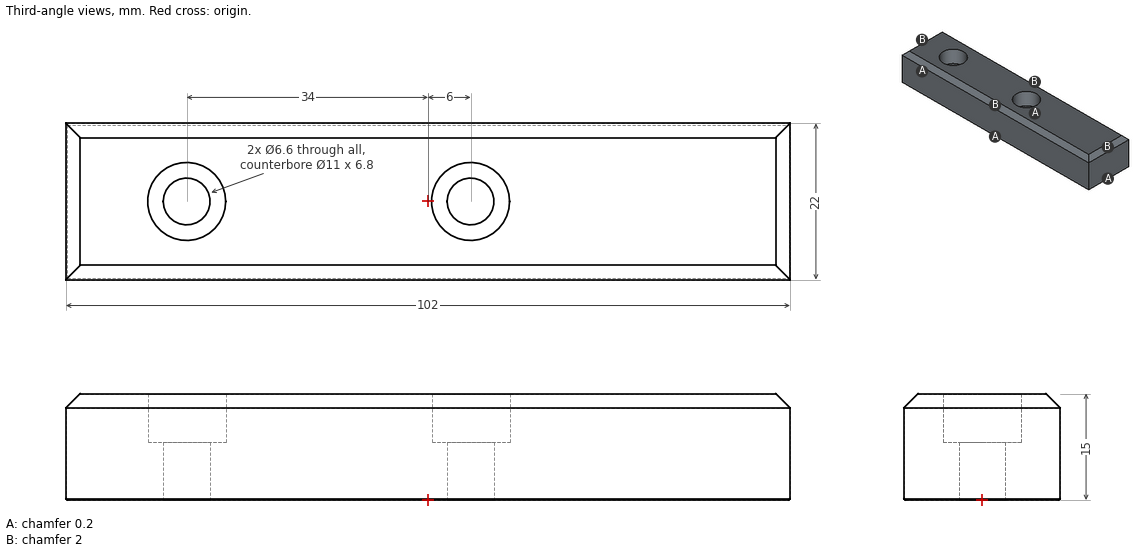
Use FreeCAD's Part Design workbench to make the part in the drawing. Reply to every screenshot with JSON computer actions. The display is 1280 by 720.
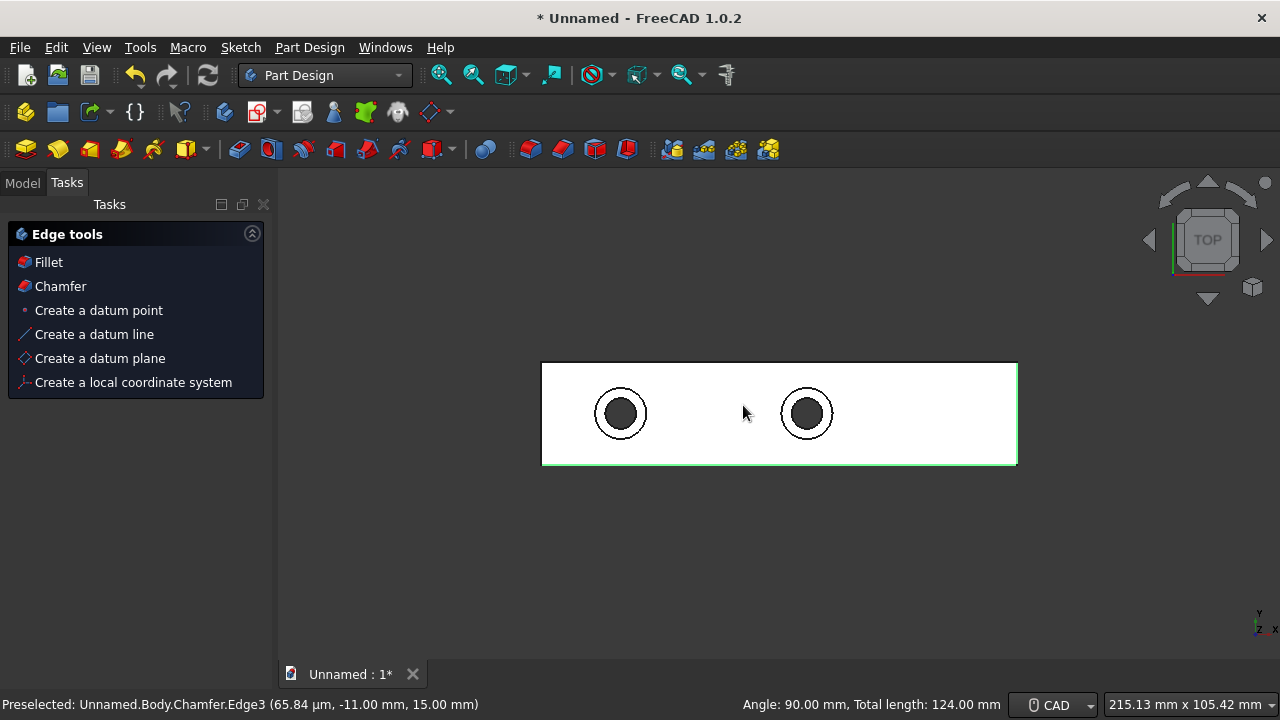
{"action": "left_click", "coordinate": [779, 361], "text": "ctrl"}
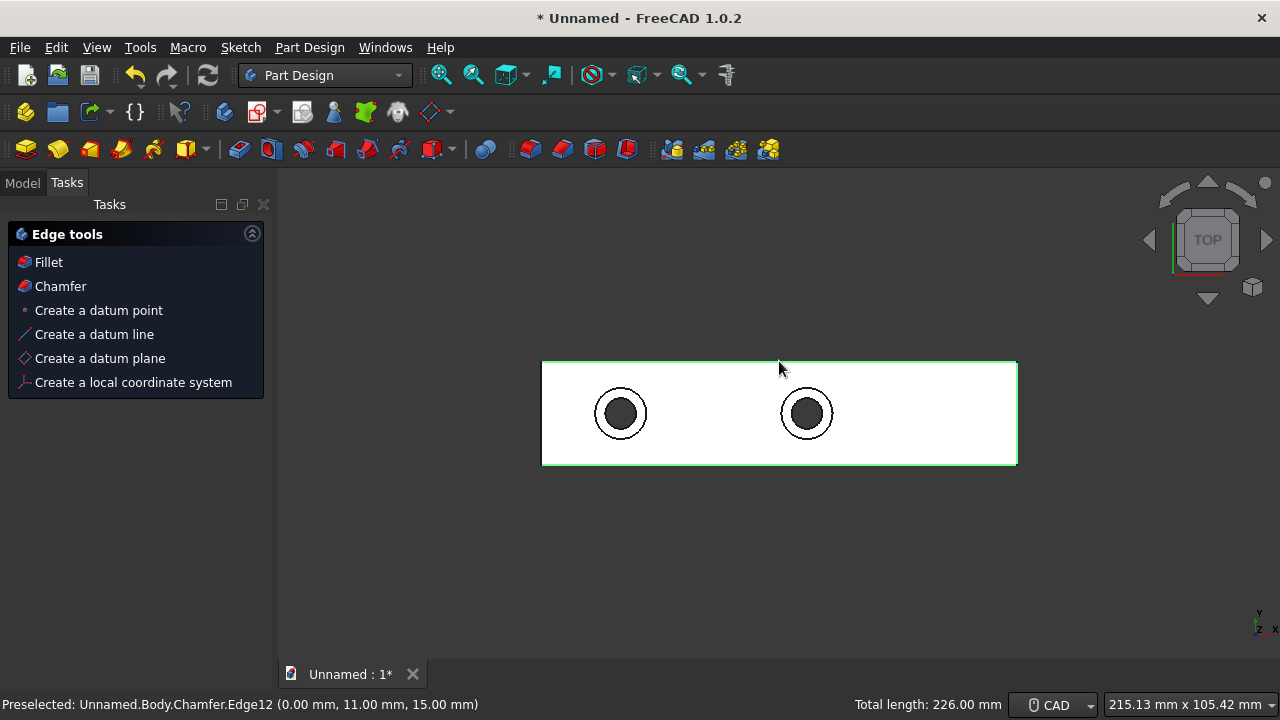
{"action": "left_click", "coordinate": [541, 413], "text": "ctrl"}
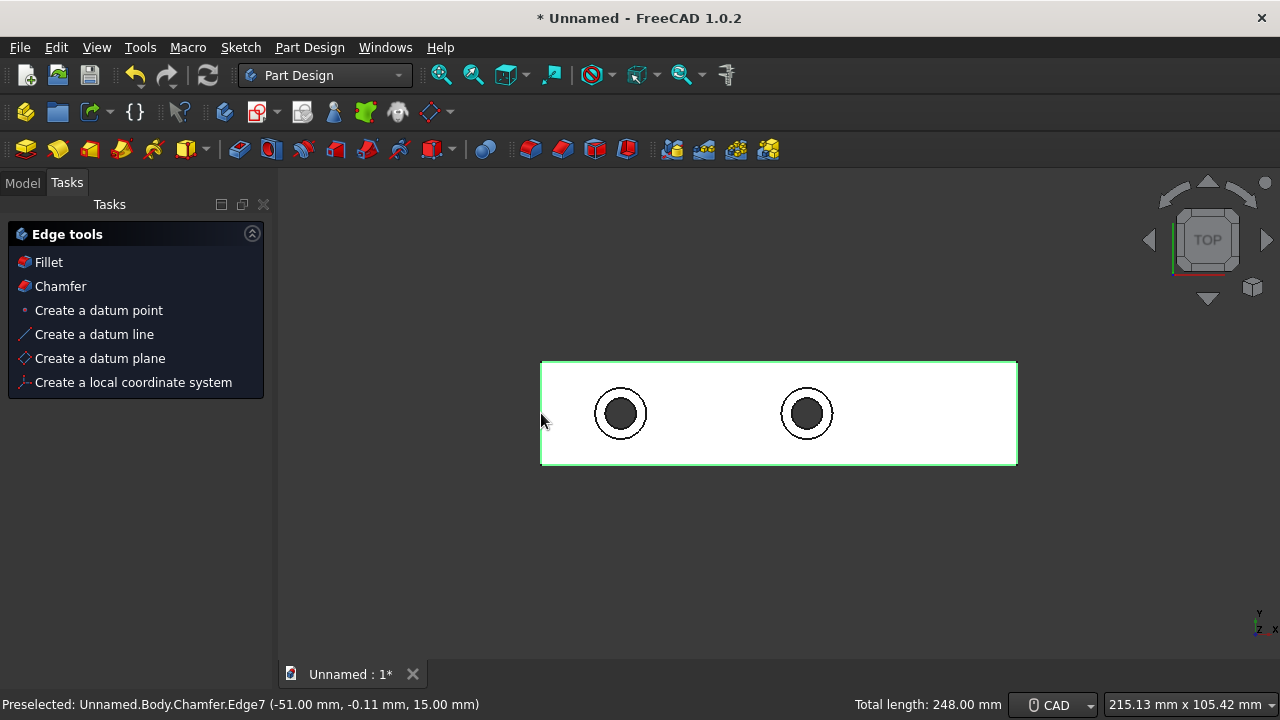
{"action": "left_click", "coordinate": [564, 150]}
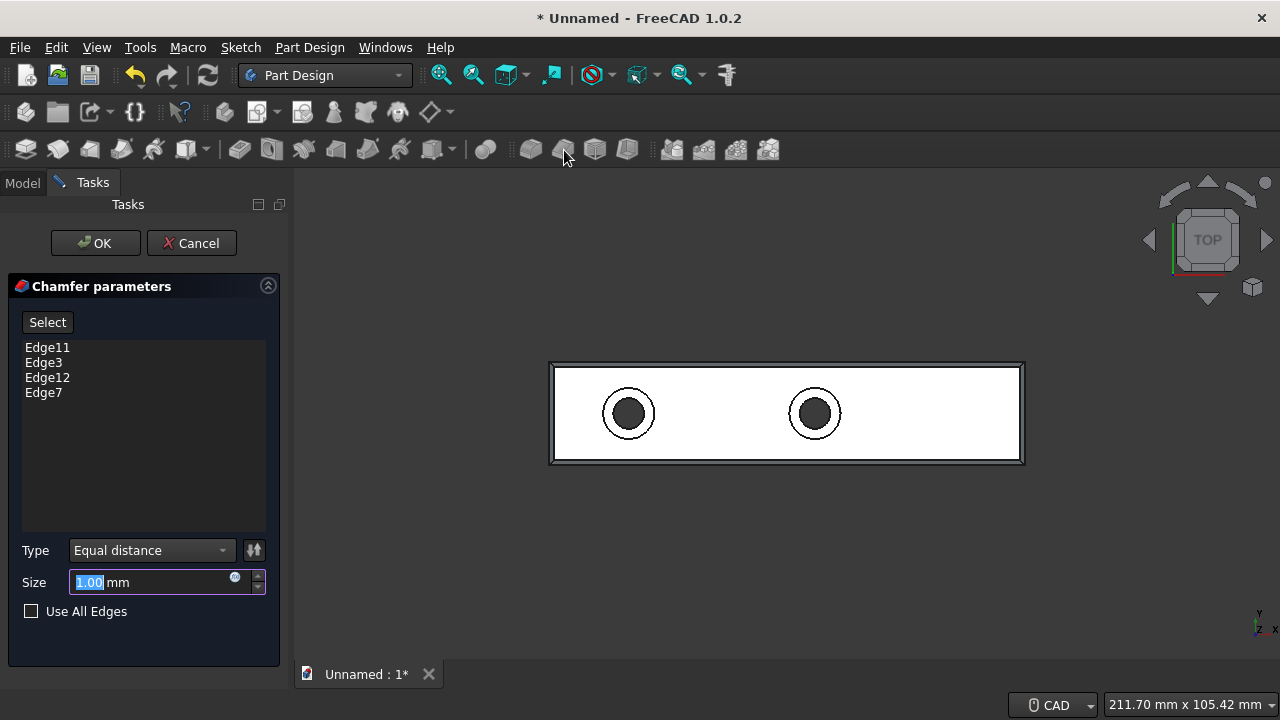
{"action": "type", "text": "2"}
{"action": "key", "text": "Tab"}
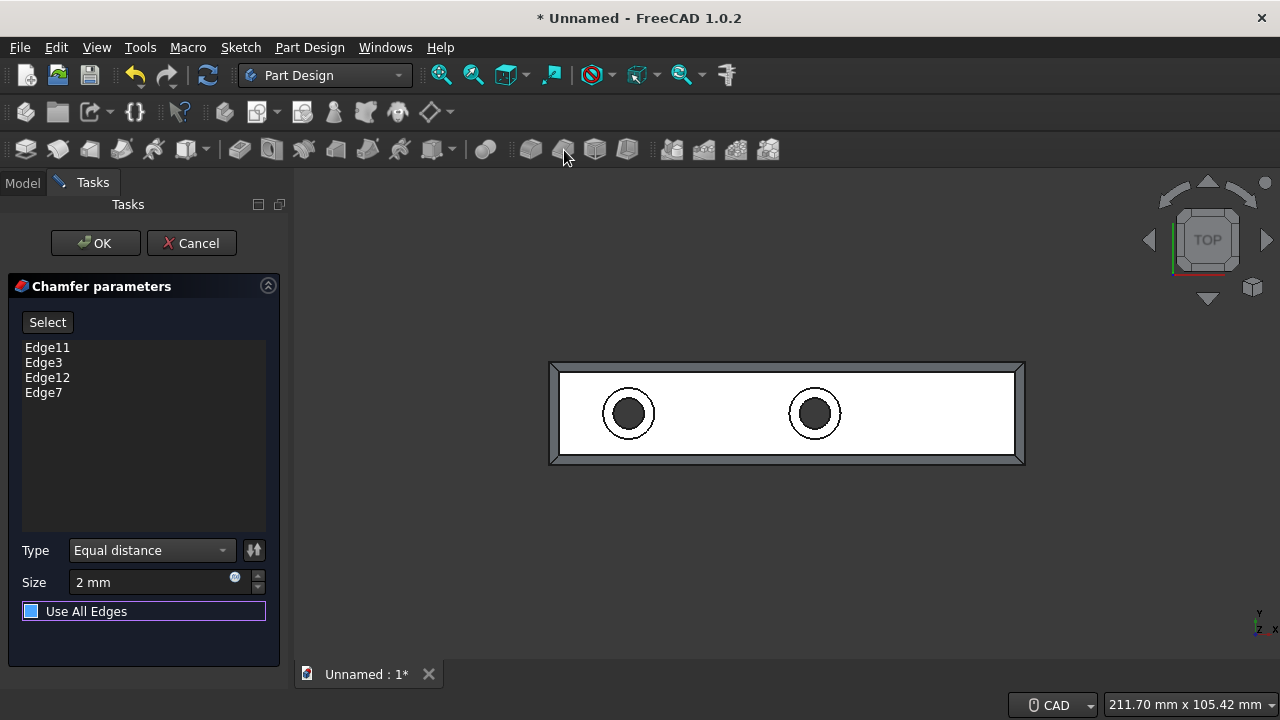
{"action": "left_click", "coordinate": [96, 243]}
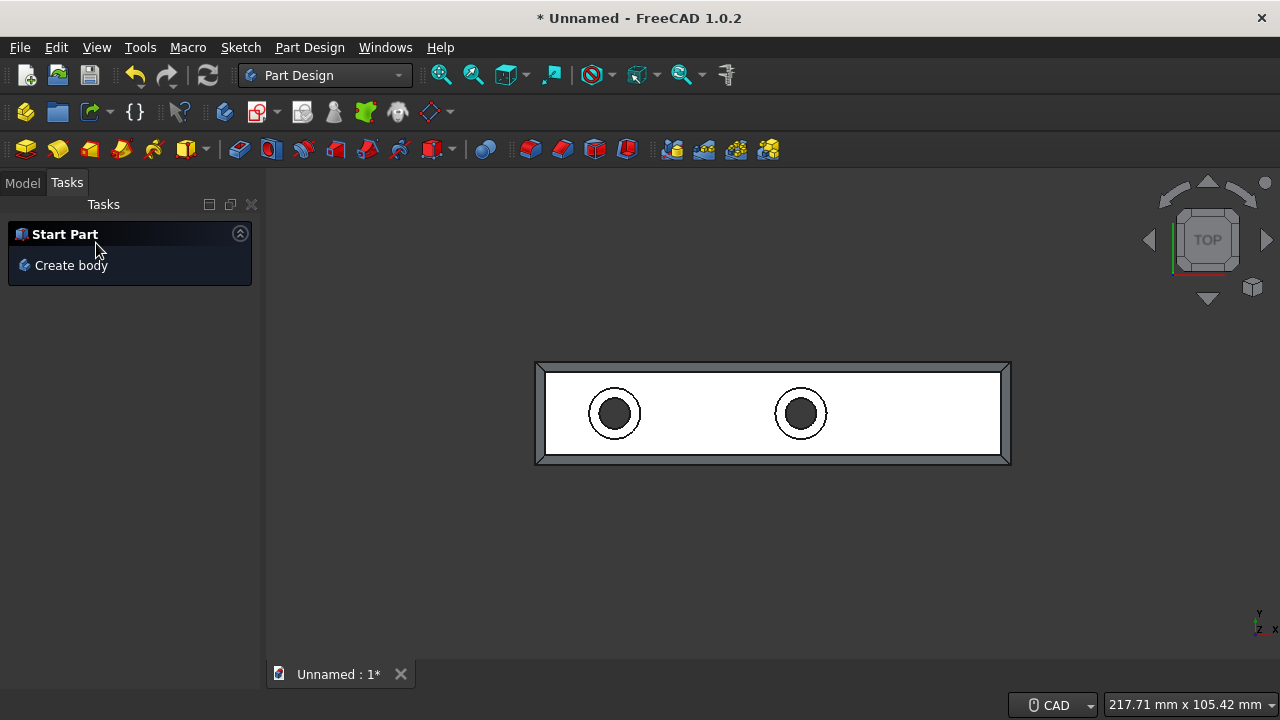
{"action": "key", "text": "0"}